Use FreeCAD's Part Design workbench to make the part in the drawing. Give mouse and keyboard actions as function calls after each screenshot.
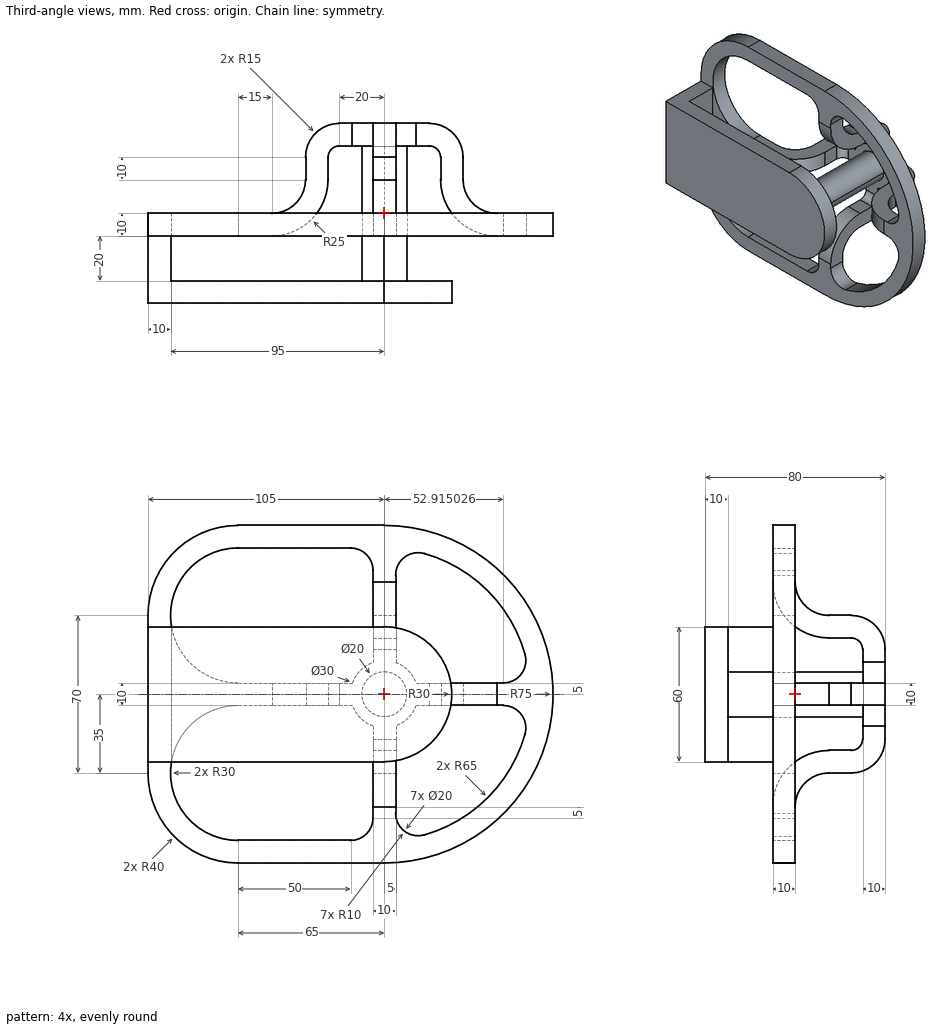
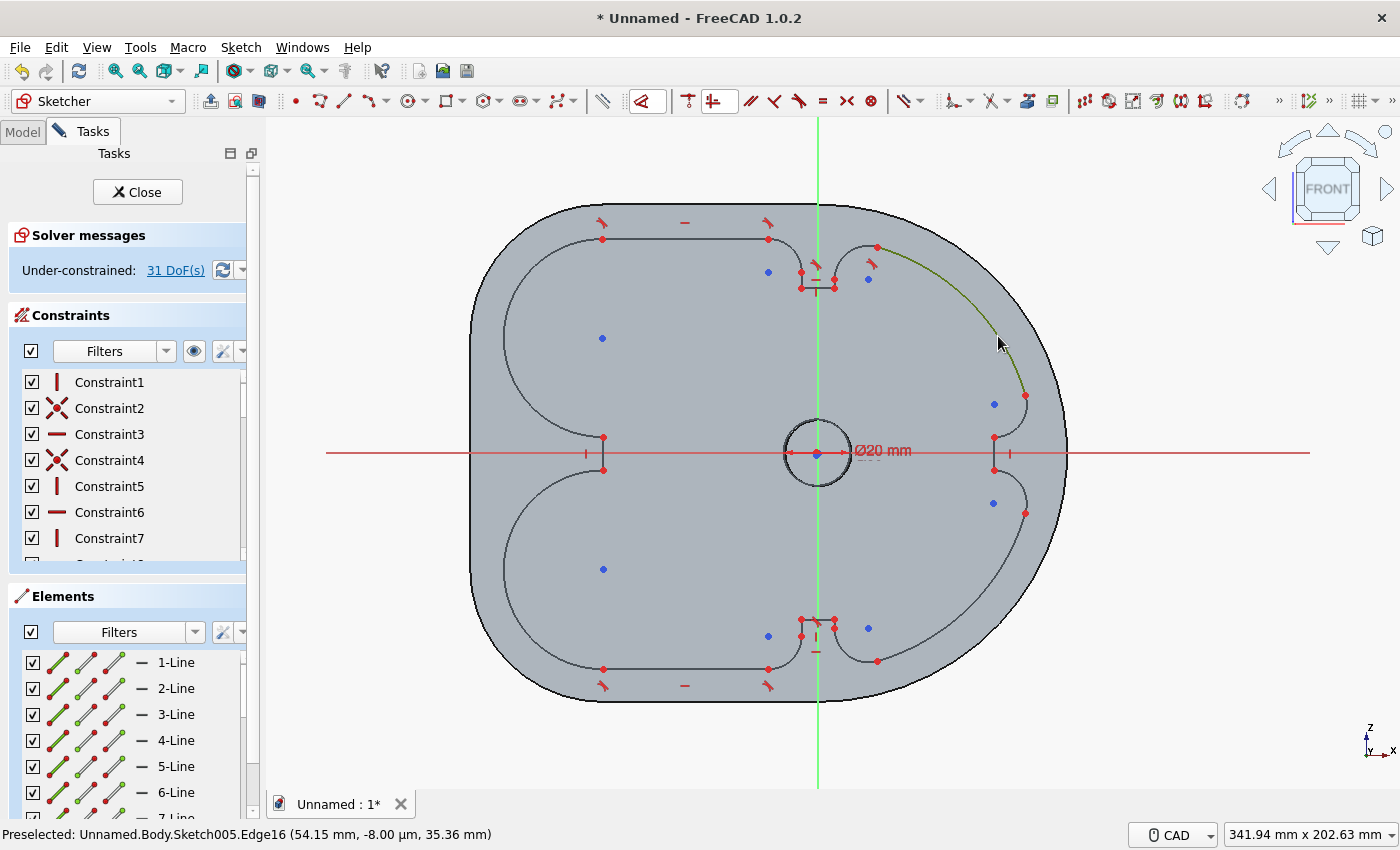
click(1012, 432)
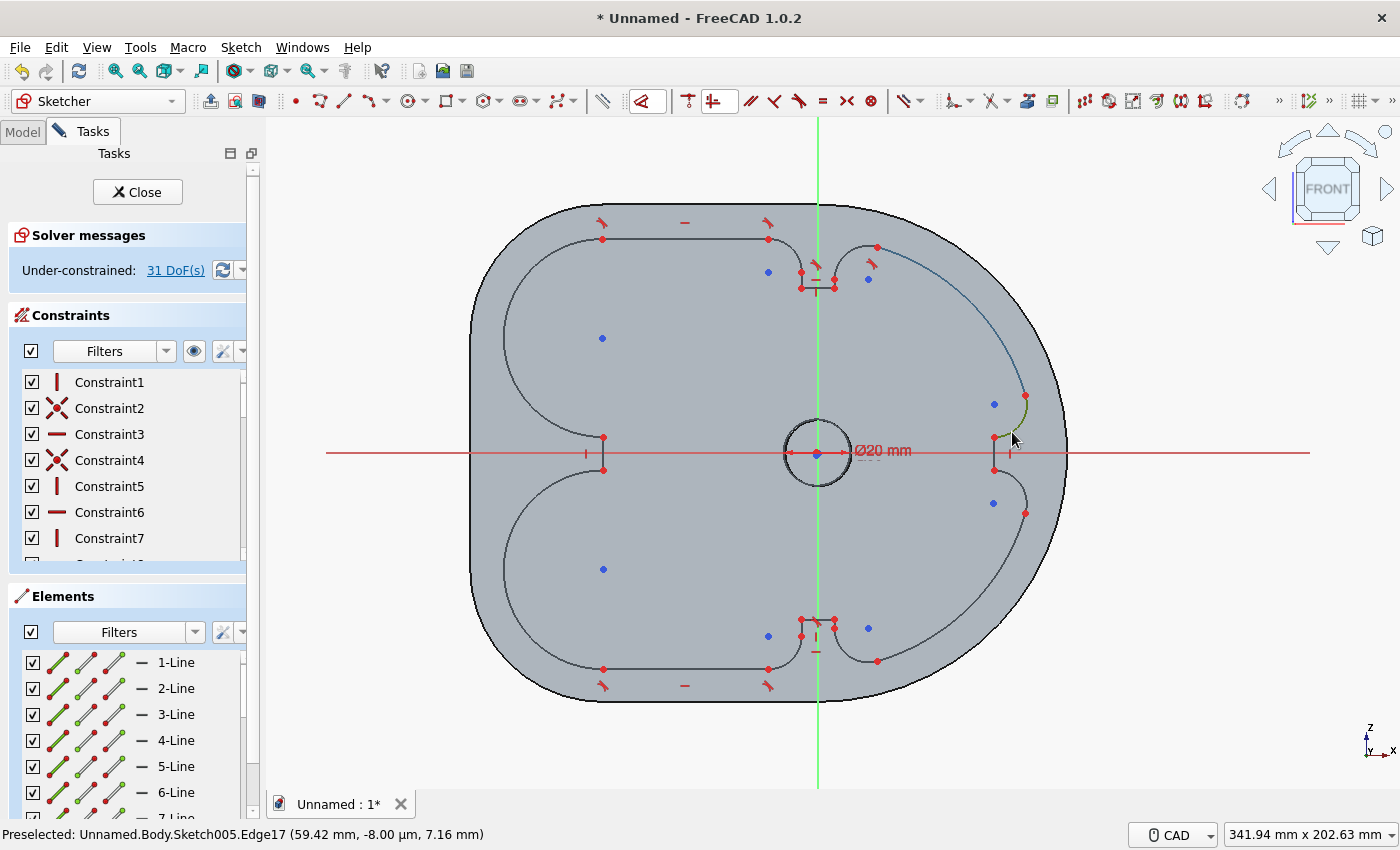
click(800, 102)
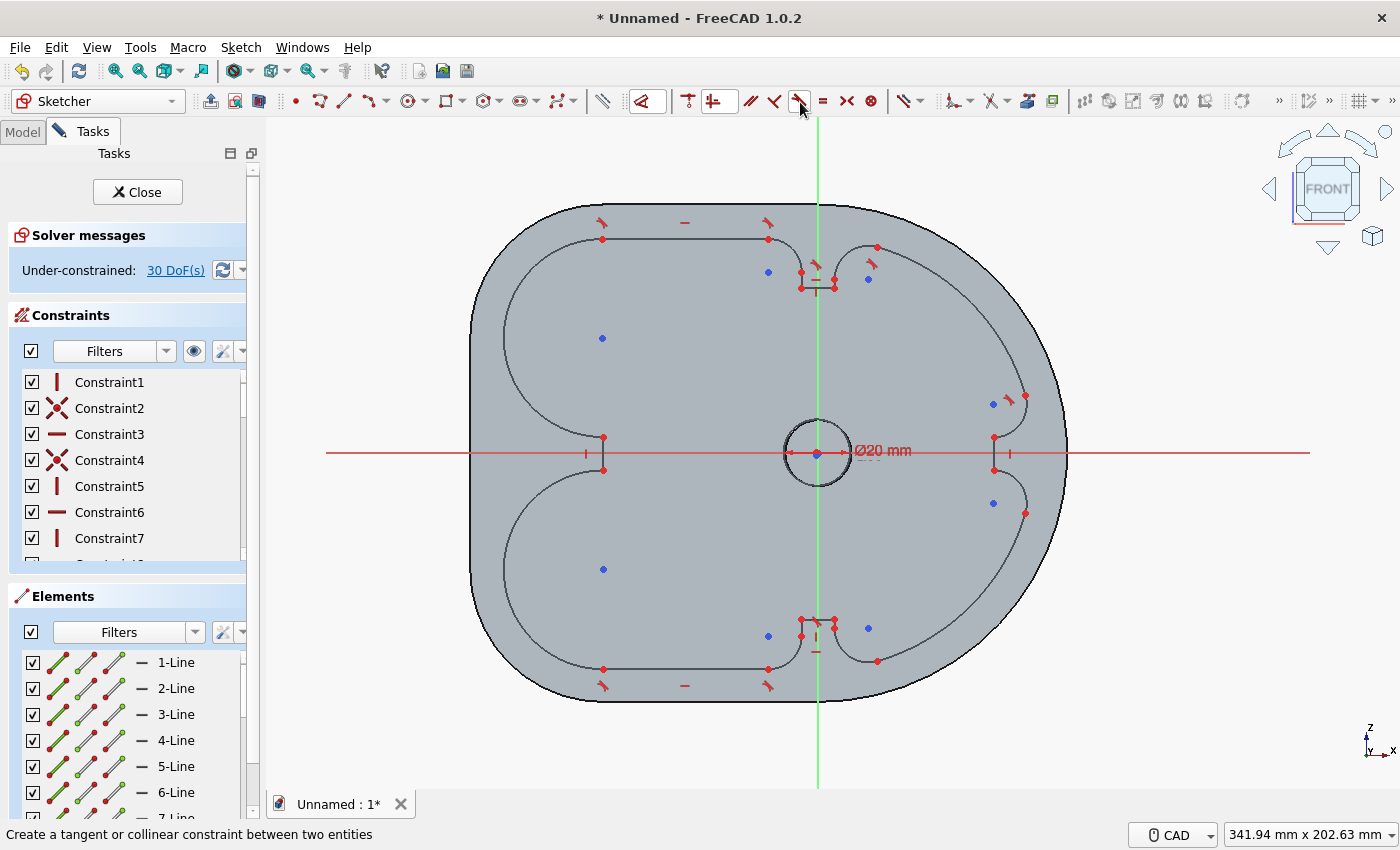
click(1026, 495)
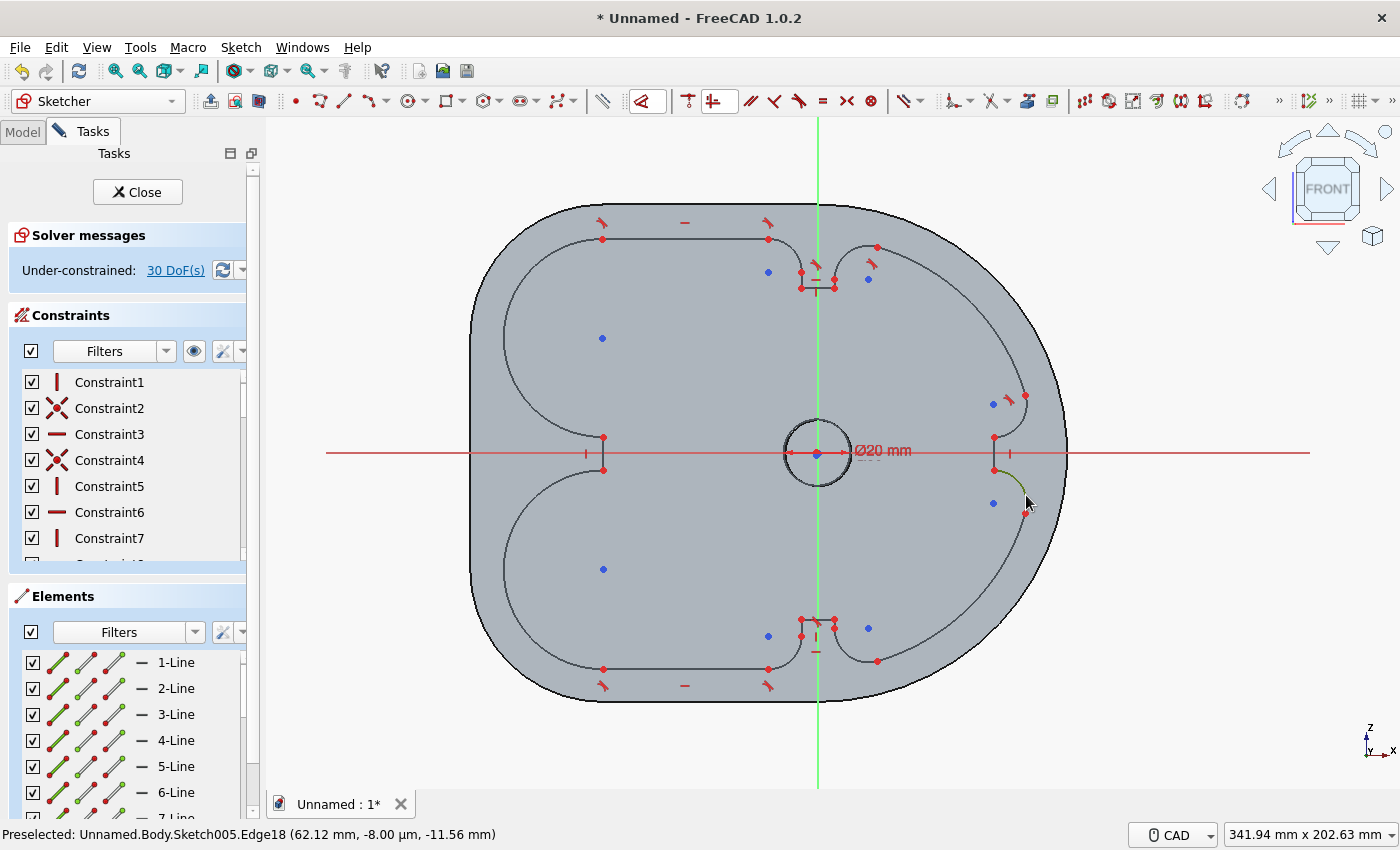
click(937, 634)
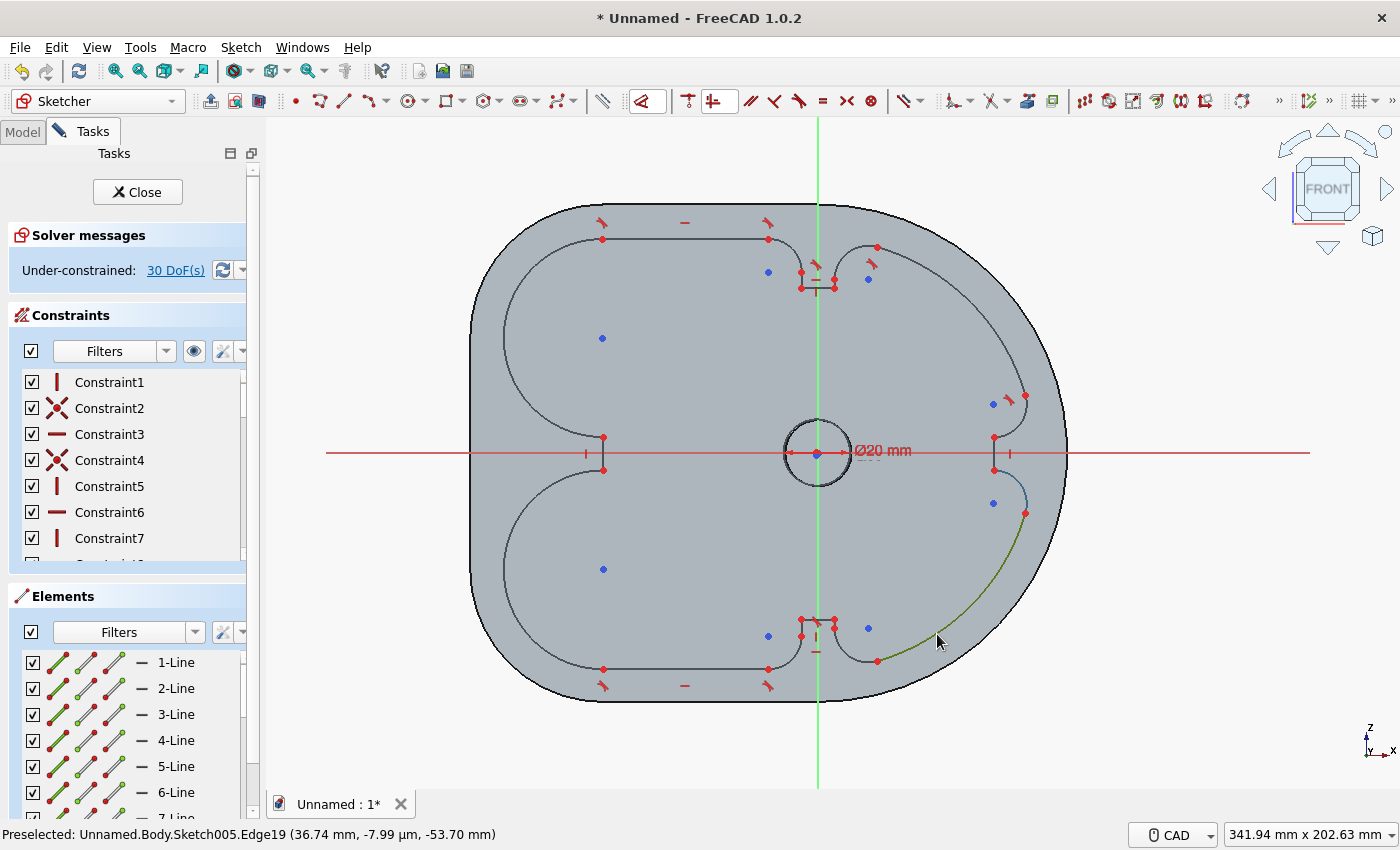
click(800, 102)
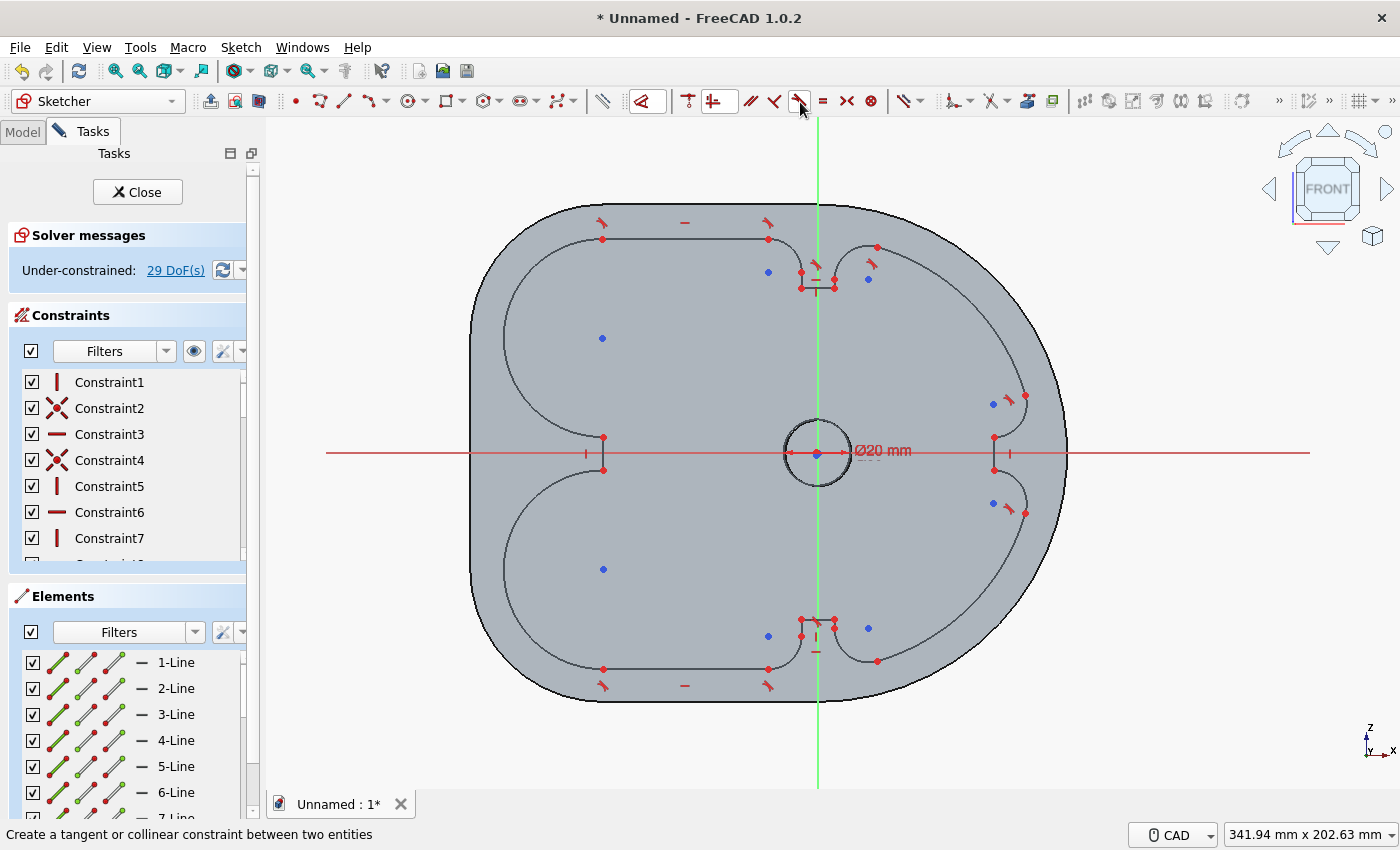
click(937, 634)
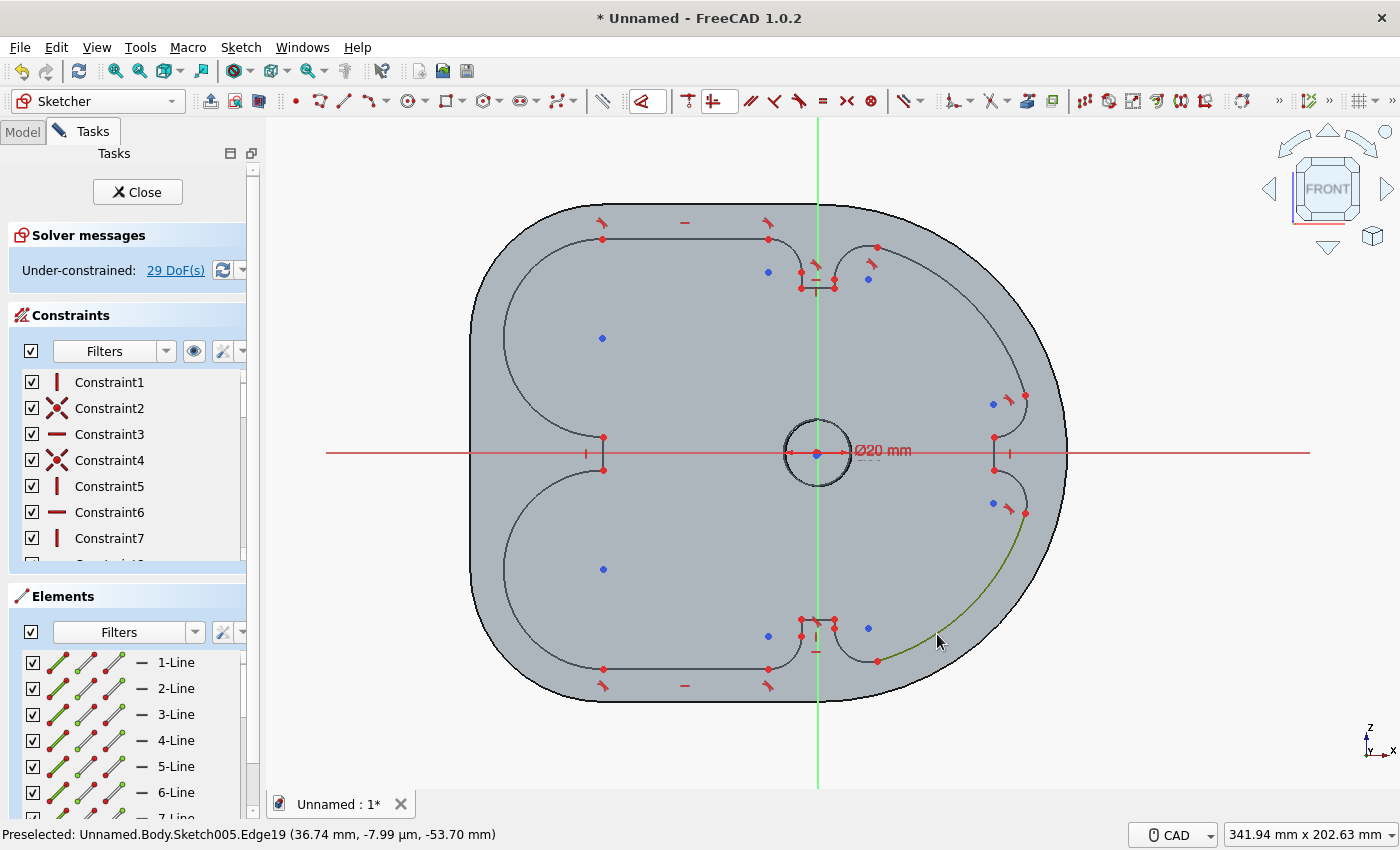
click(840, 646)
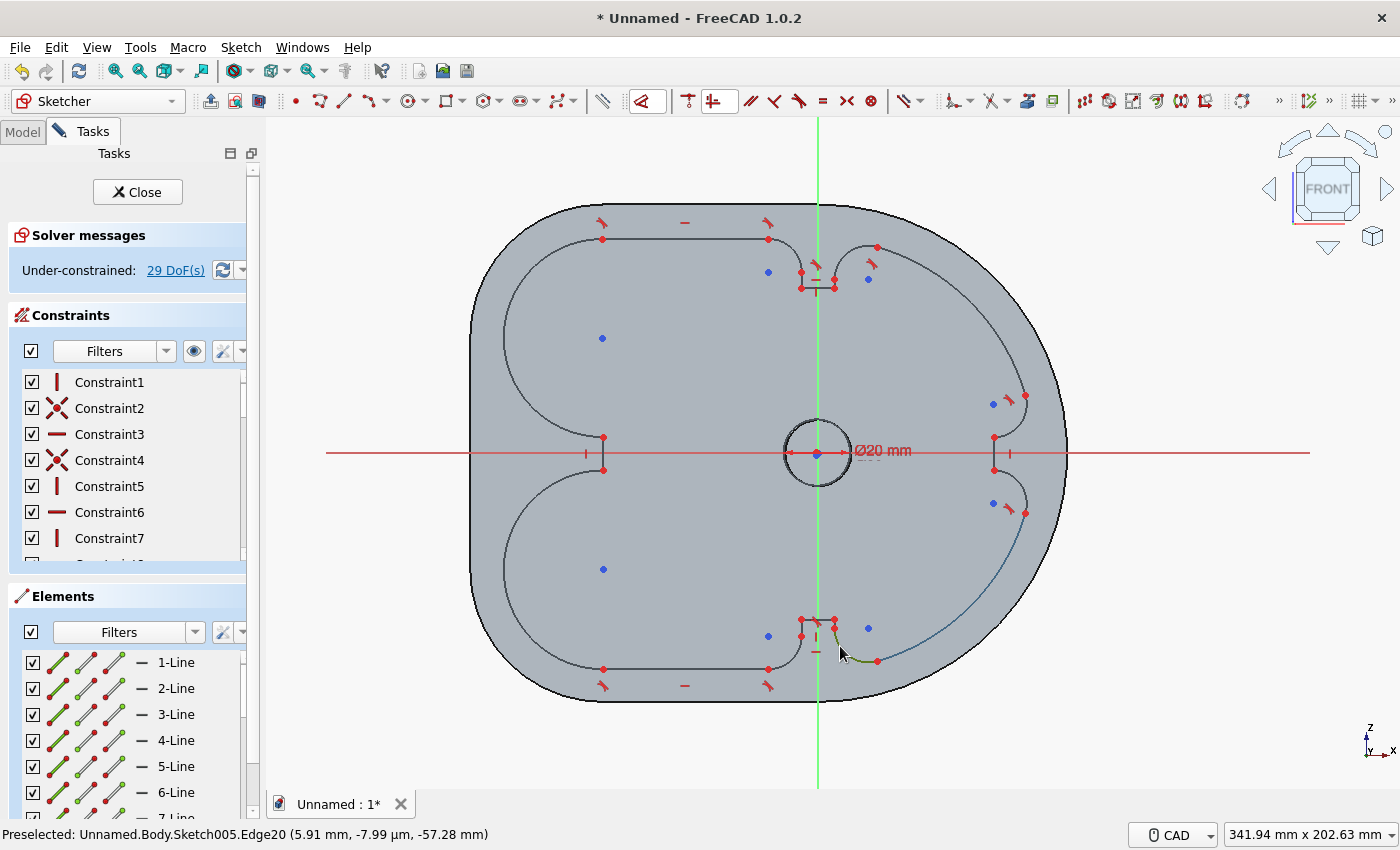
click(800, 102)